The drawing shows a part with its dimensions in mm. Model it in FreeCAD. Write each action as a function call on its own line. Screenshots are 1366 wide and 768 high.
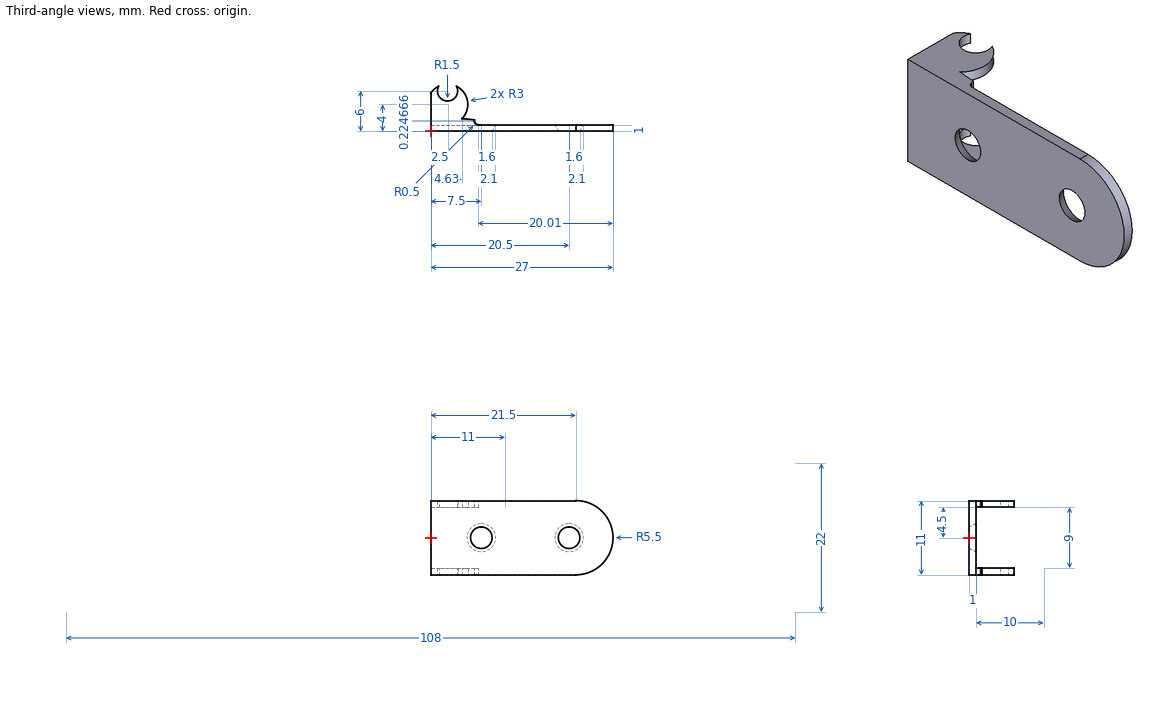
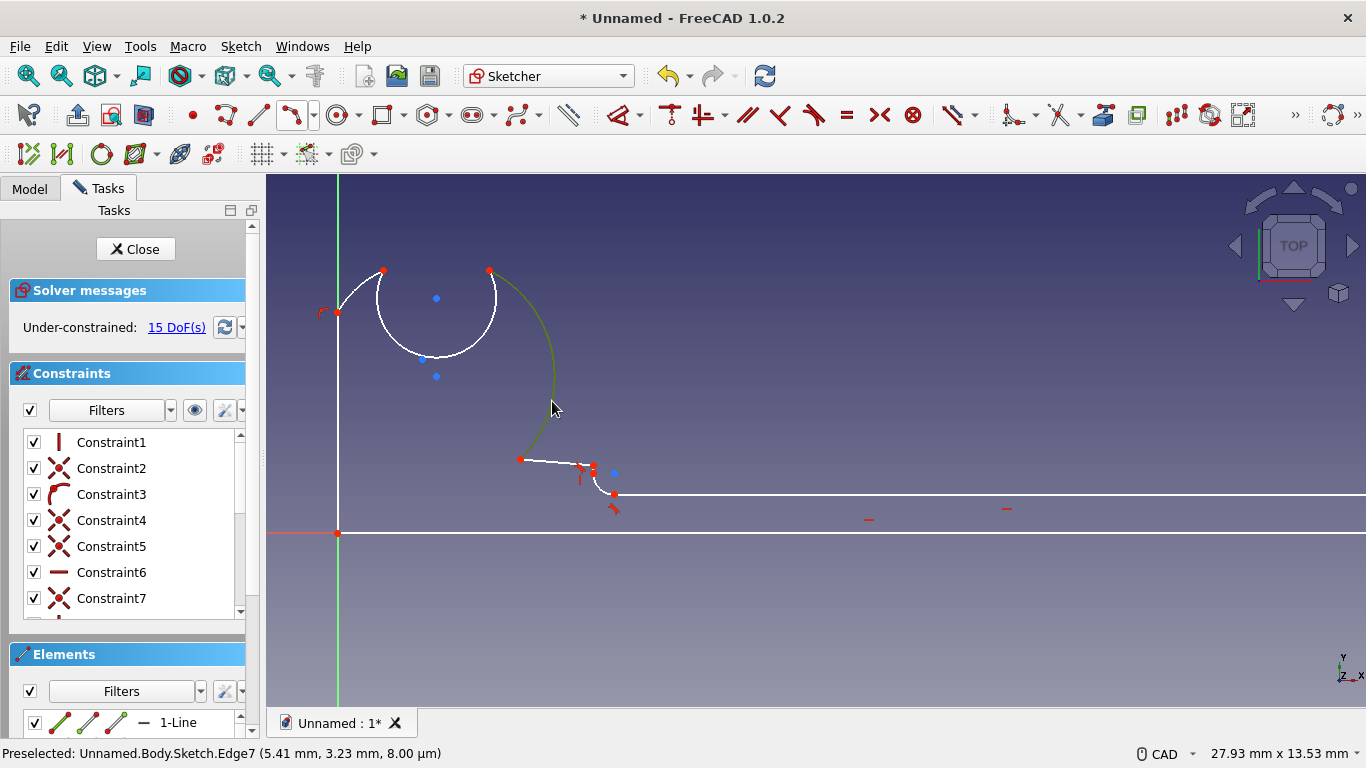
click(367, 280)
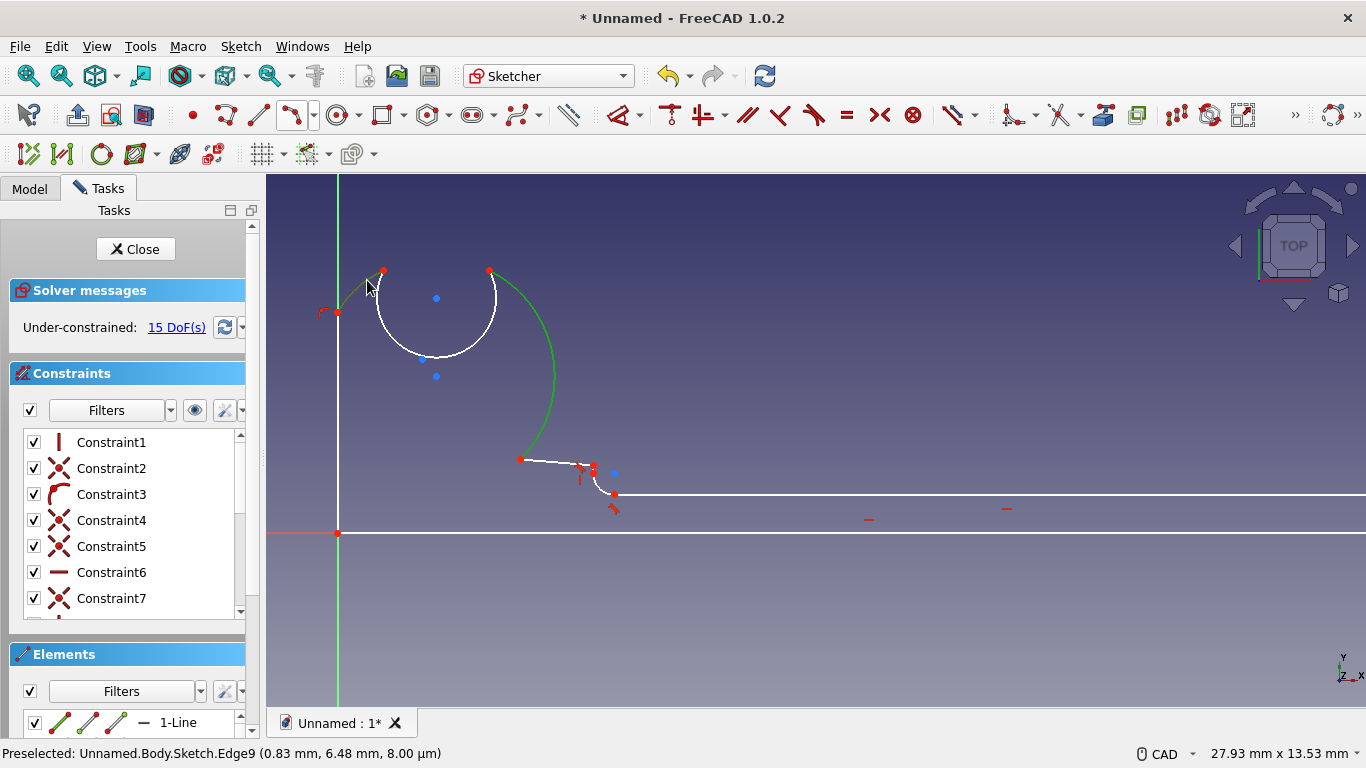
key(c)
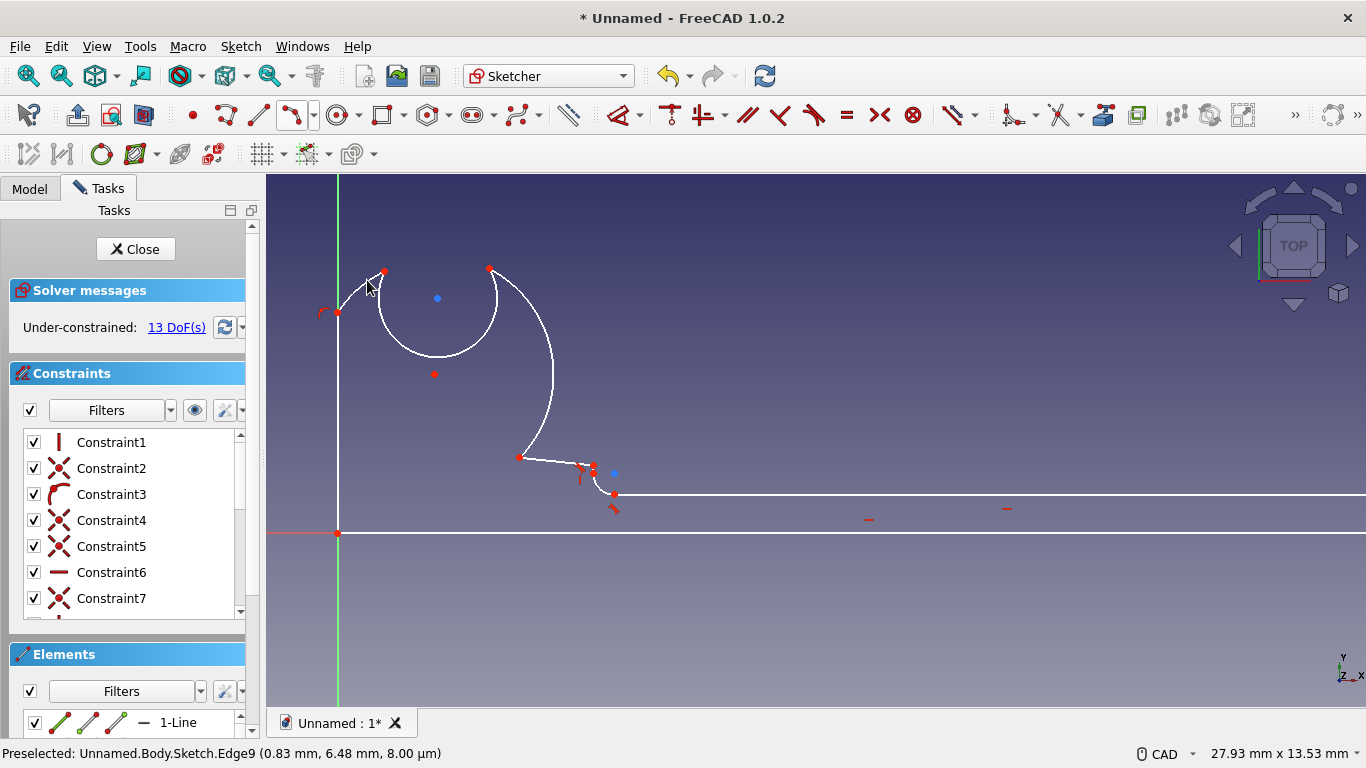
click(551, 400)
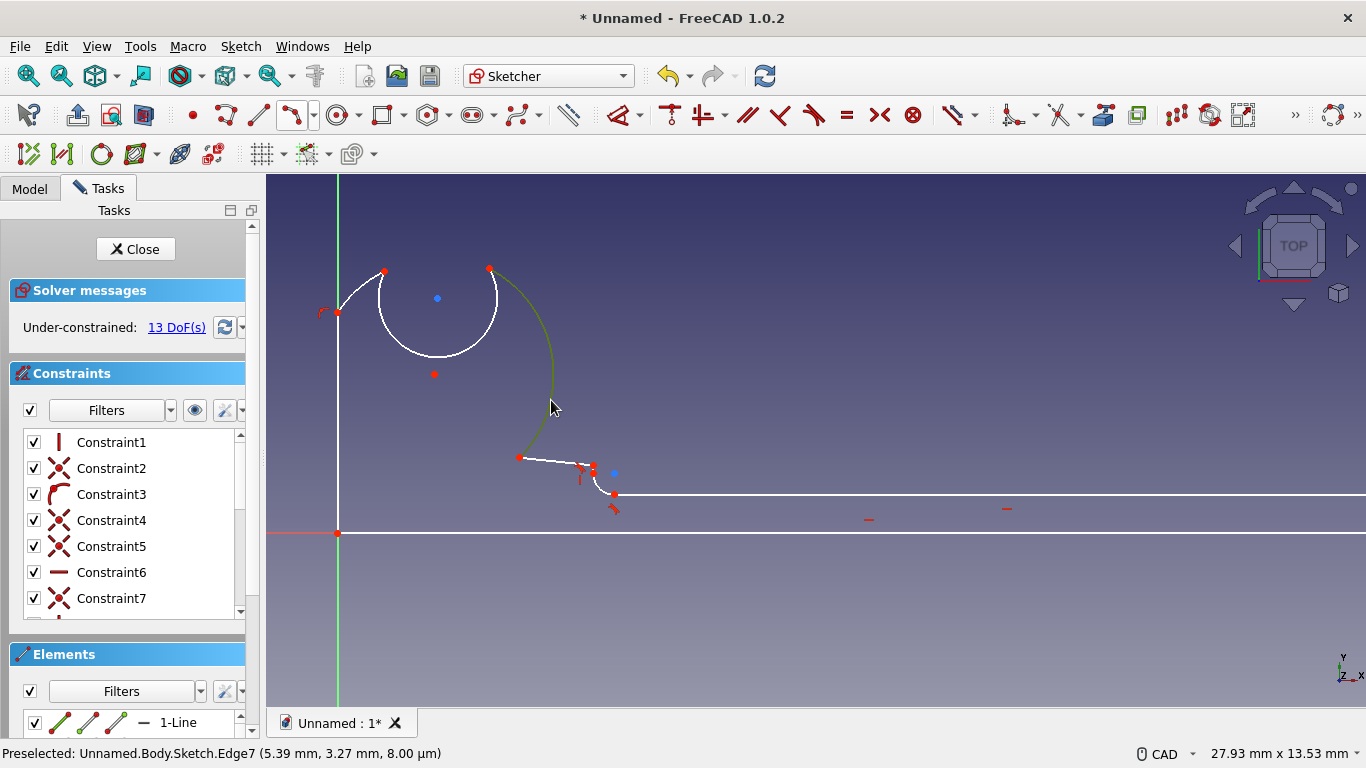
click(368, 281)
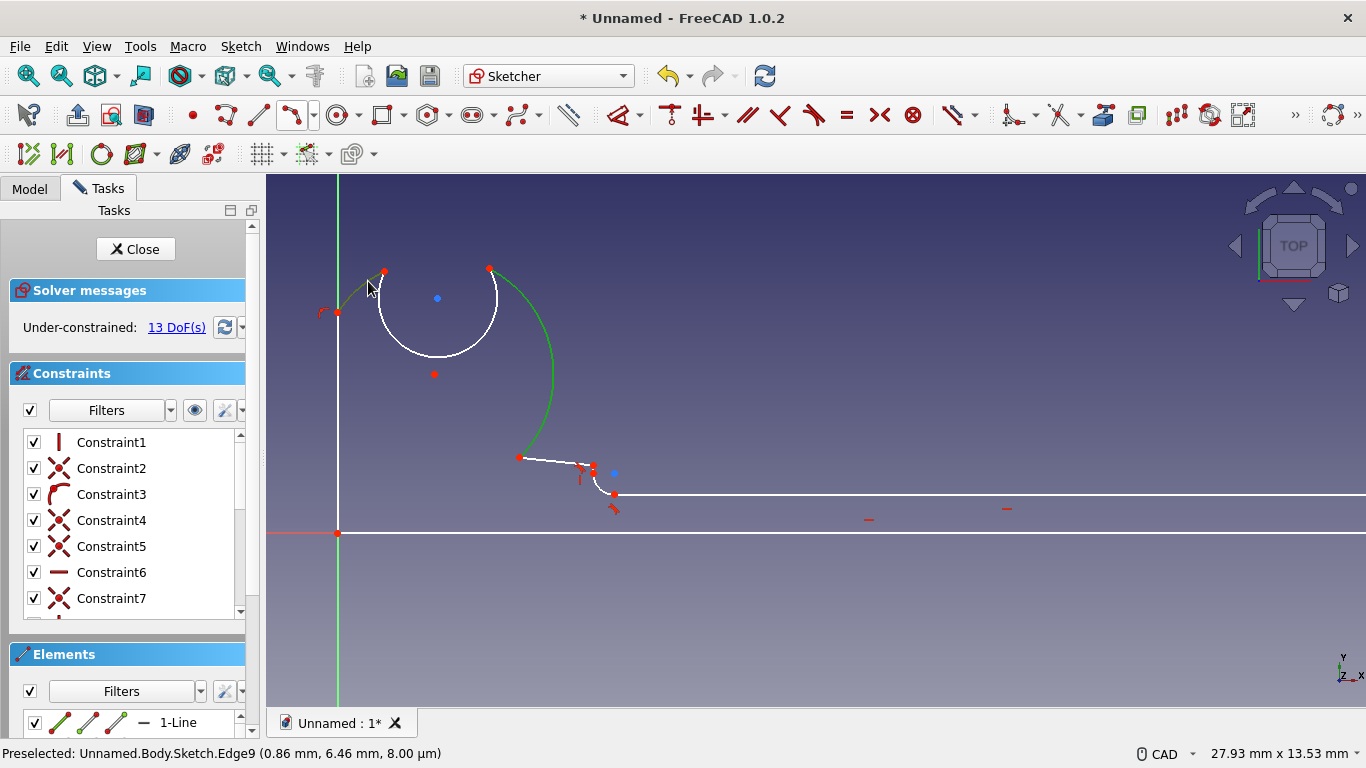
key(e)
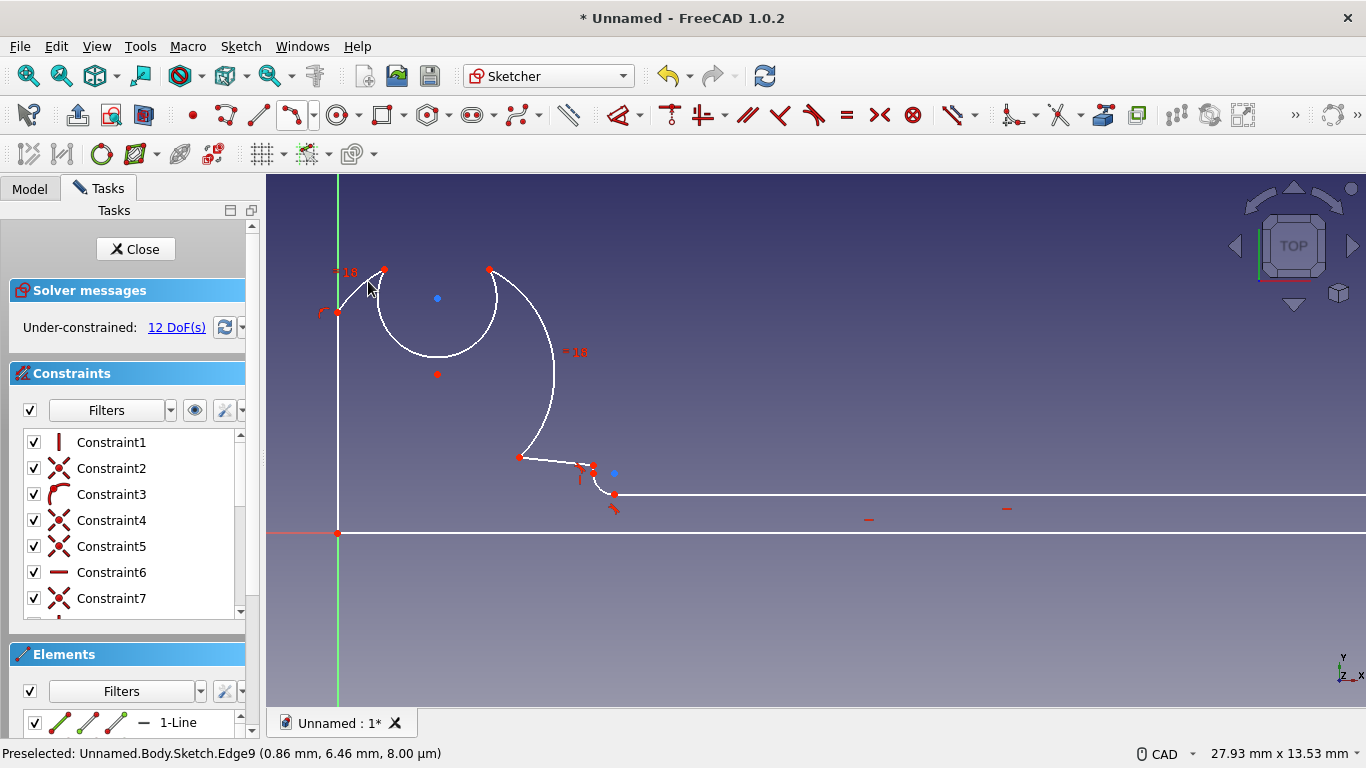
click(552, 400)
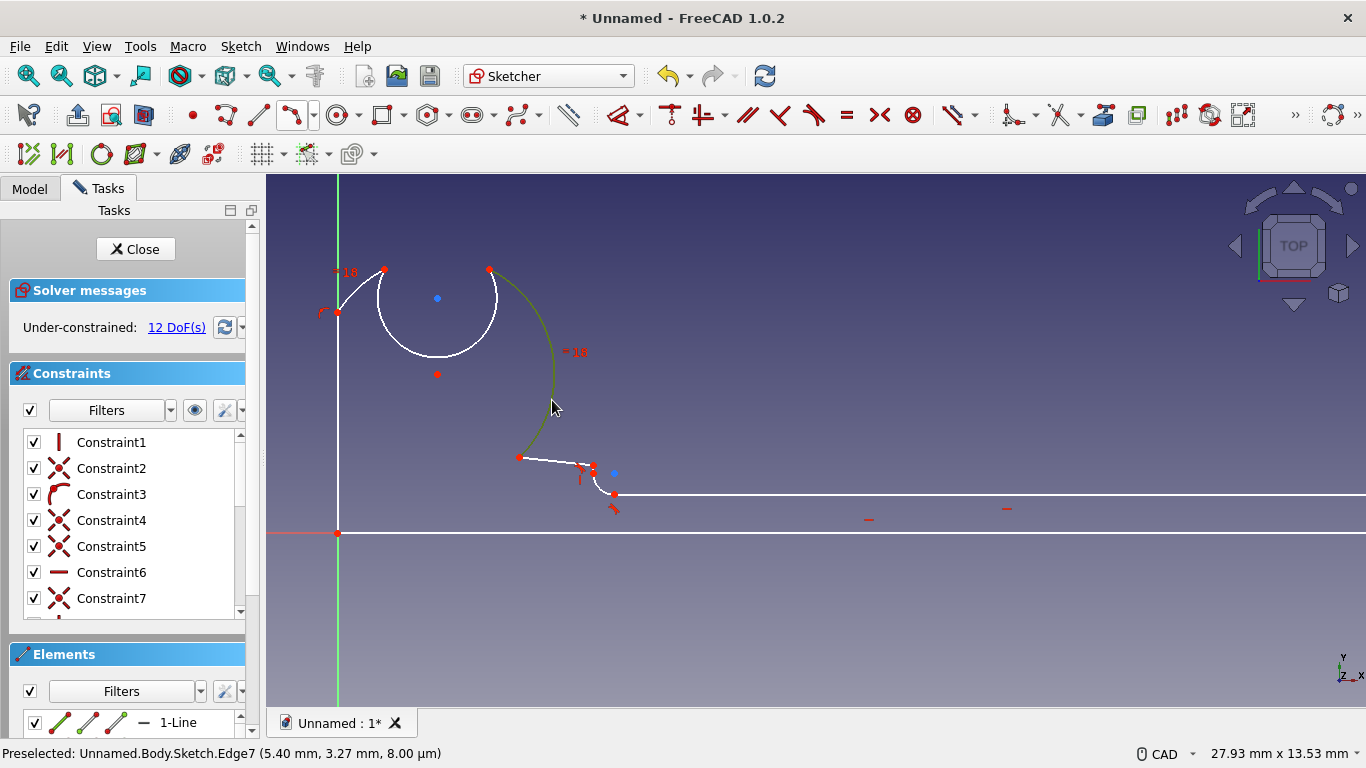
key(k)
key(r)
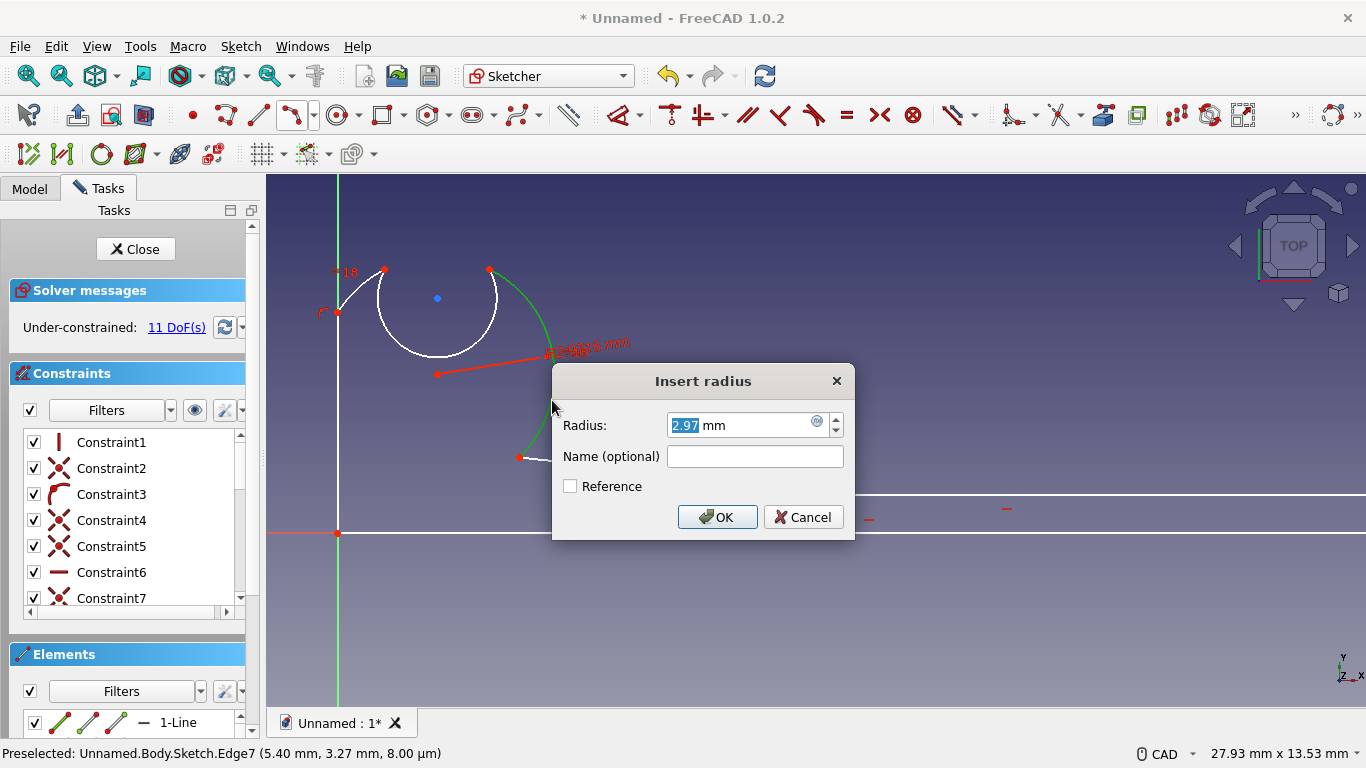
text(3)
key(Return)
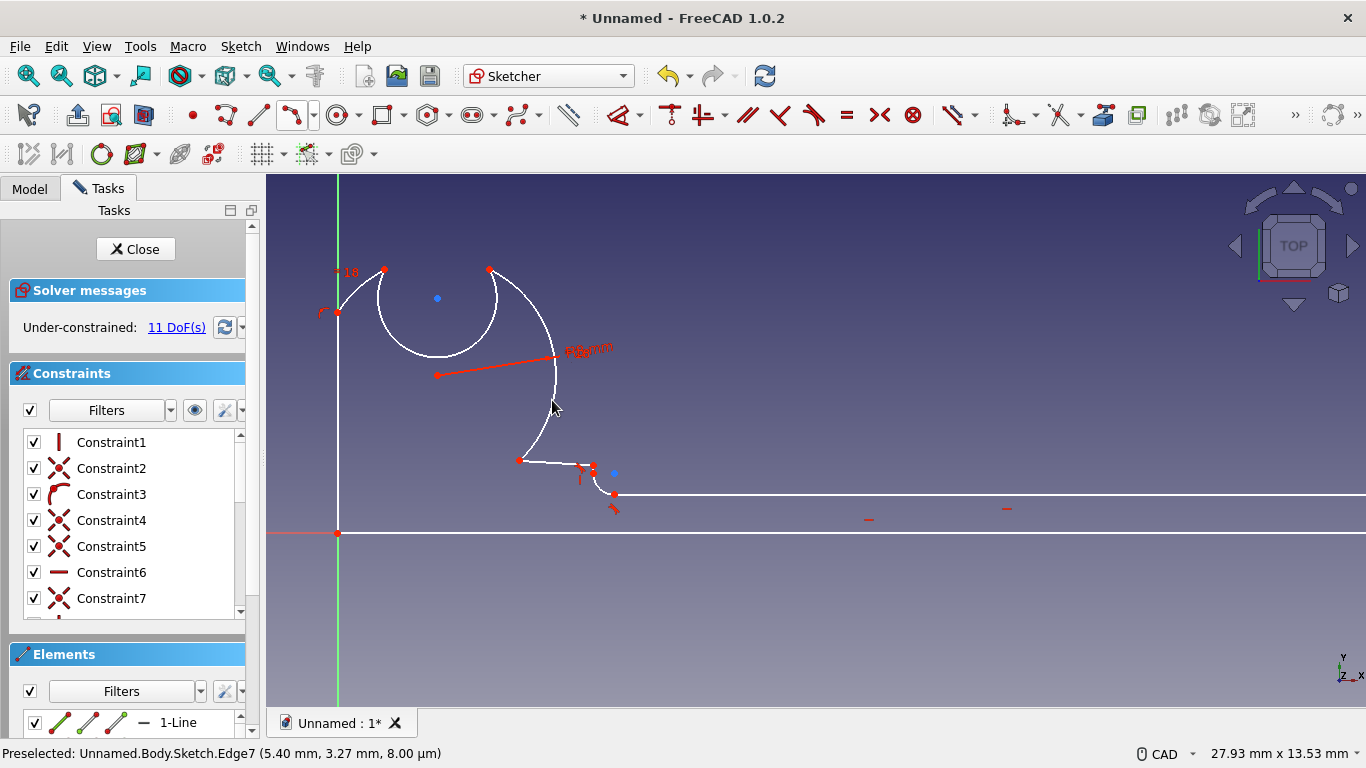
click(394, 338)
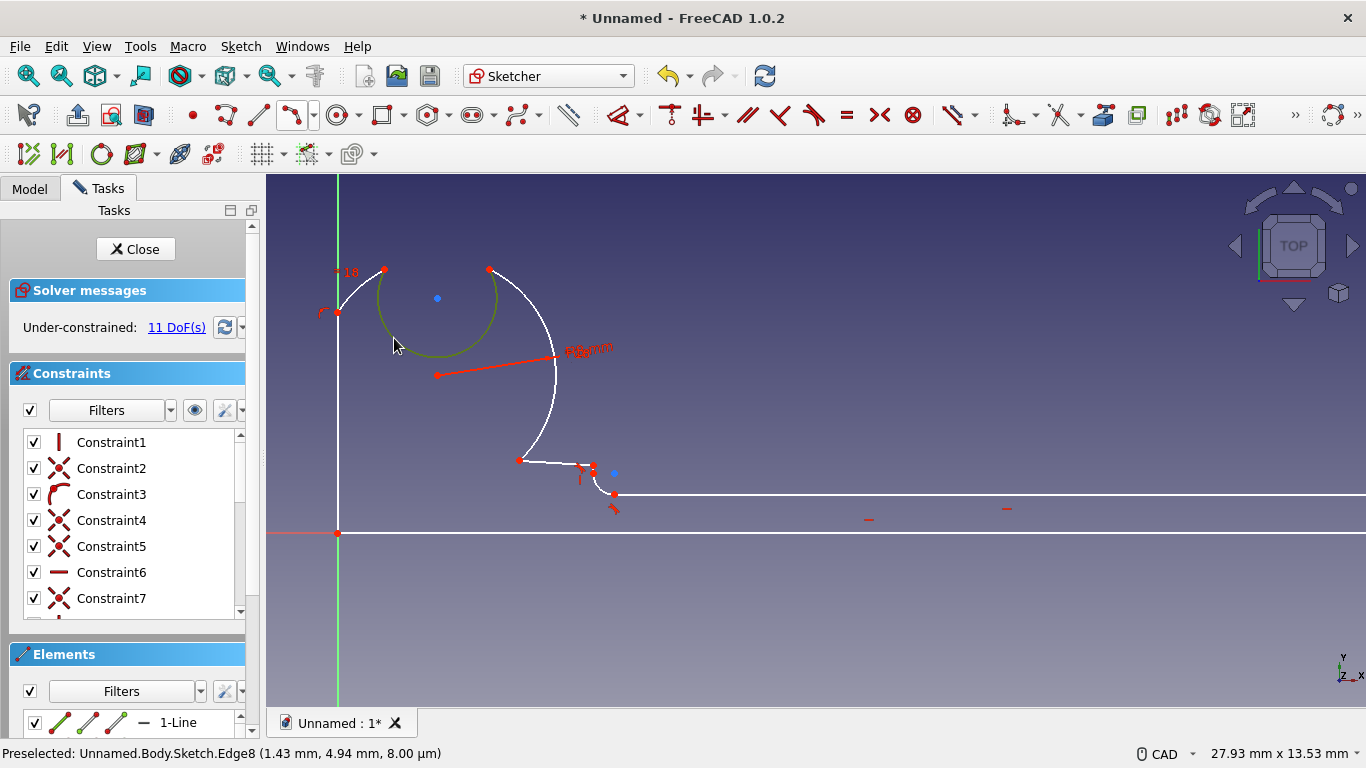
key(k)
key(r)